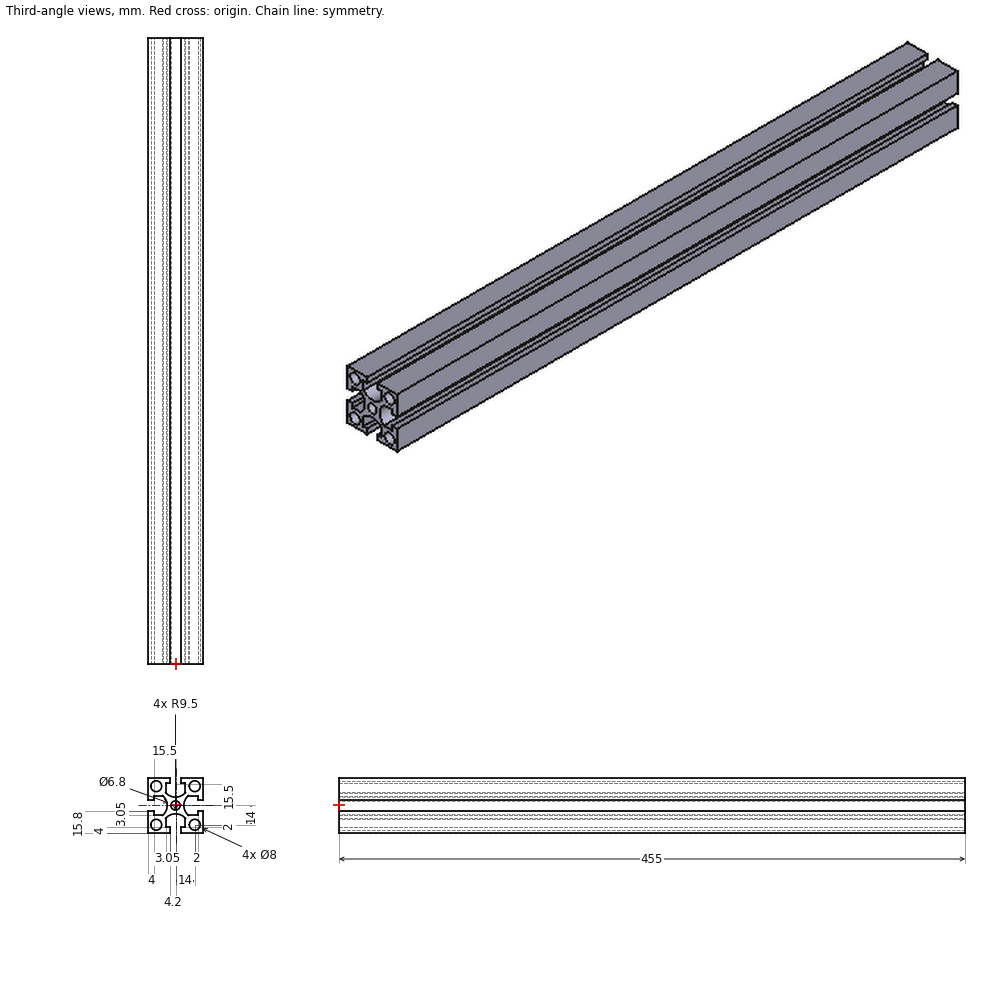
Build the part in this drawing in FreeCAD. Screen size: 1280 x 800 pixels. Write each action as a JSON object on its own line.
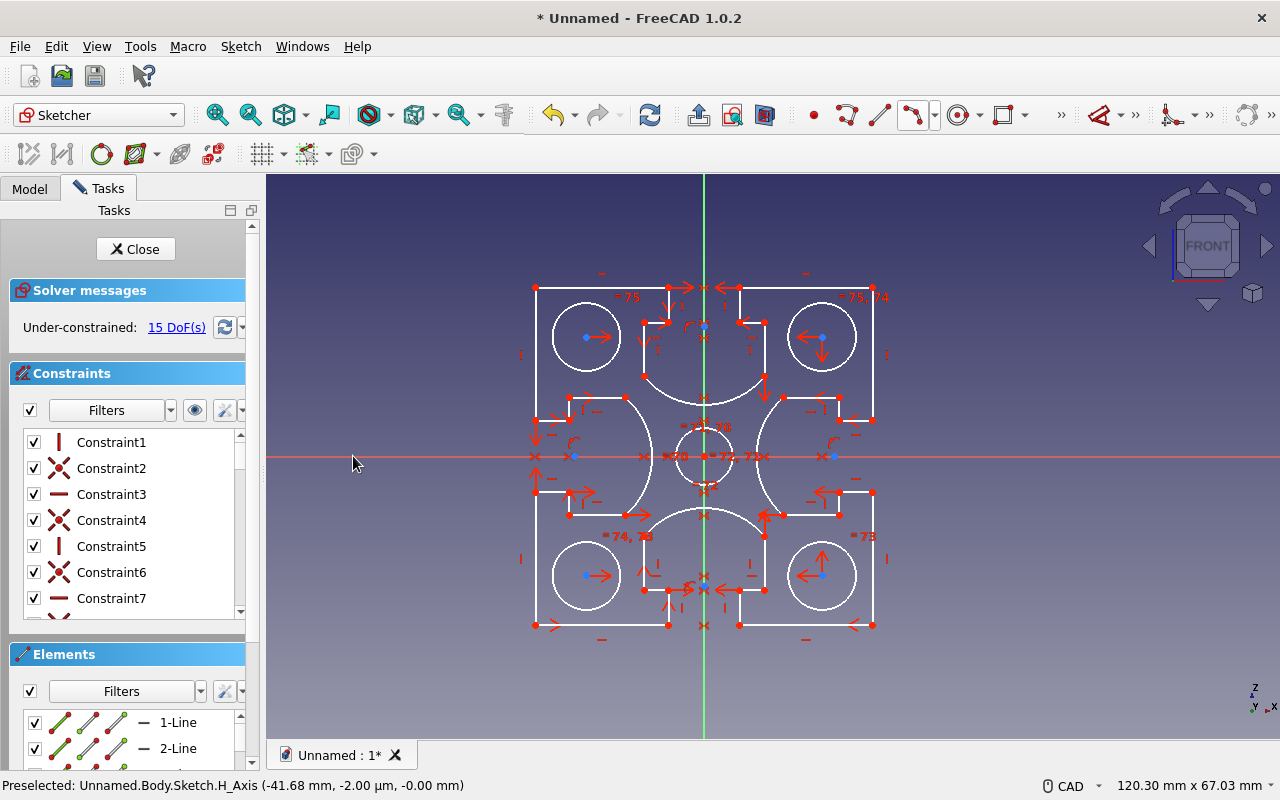
{"action": "left_click", "coordinate": [1098, 116]}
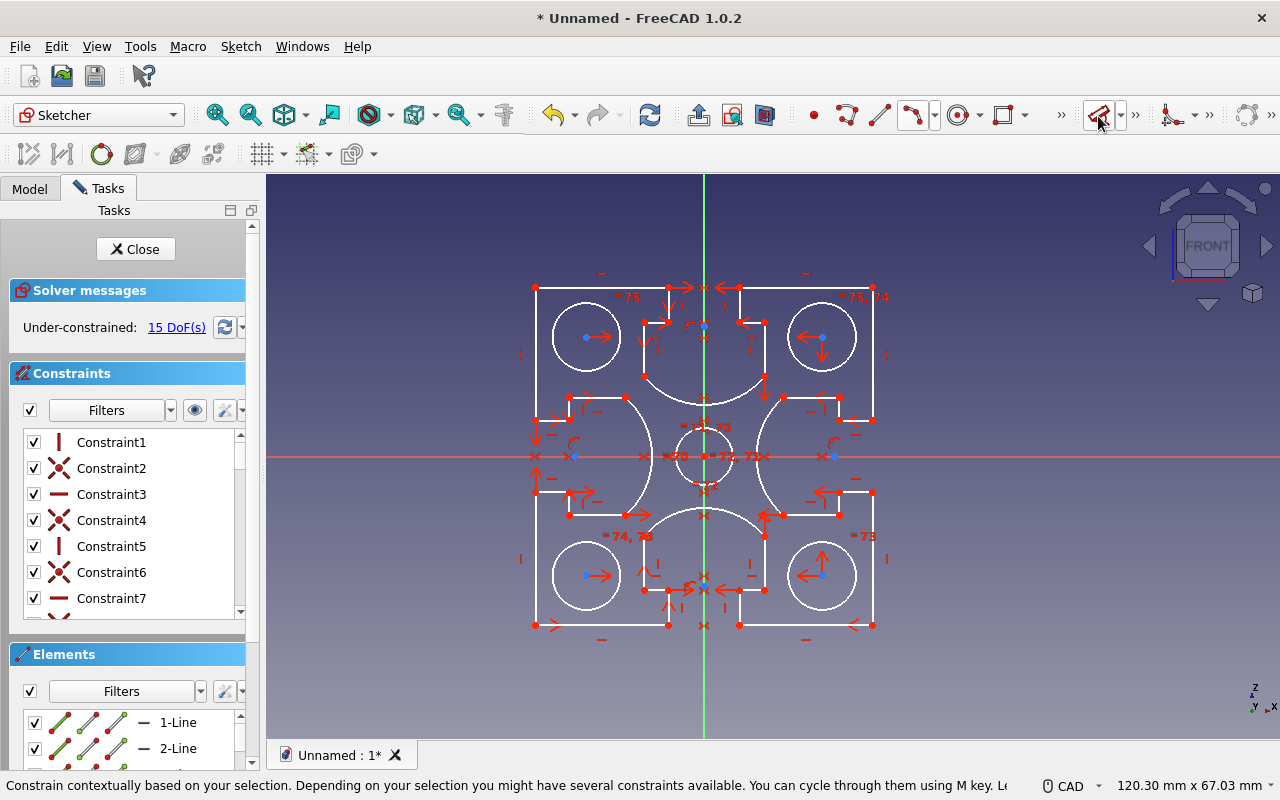
{"action": "left_click", "coordinate": [648, 483]}
{"action": "left_click", "coordinate": [678, 494]}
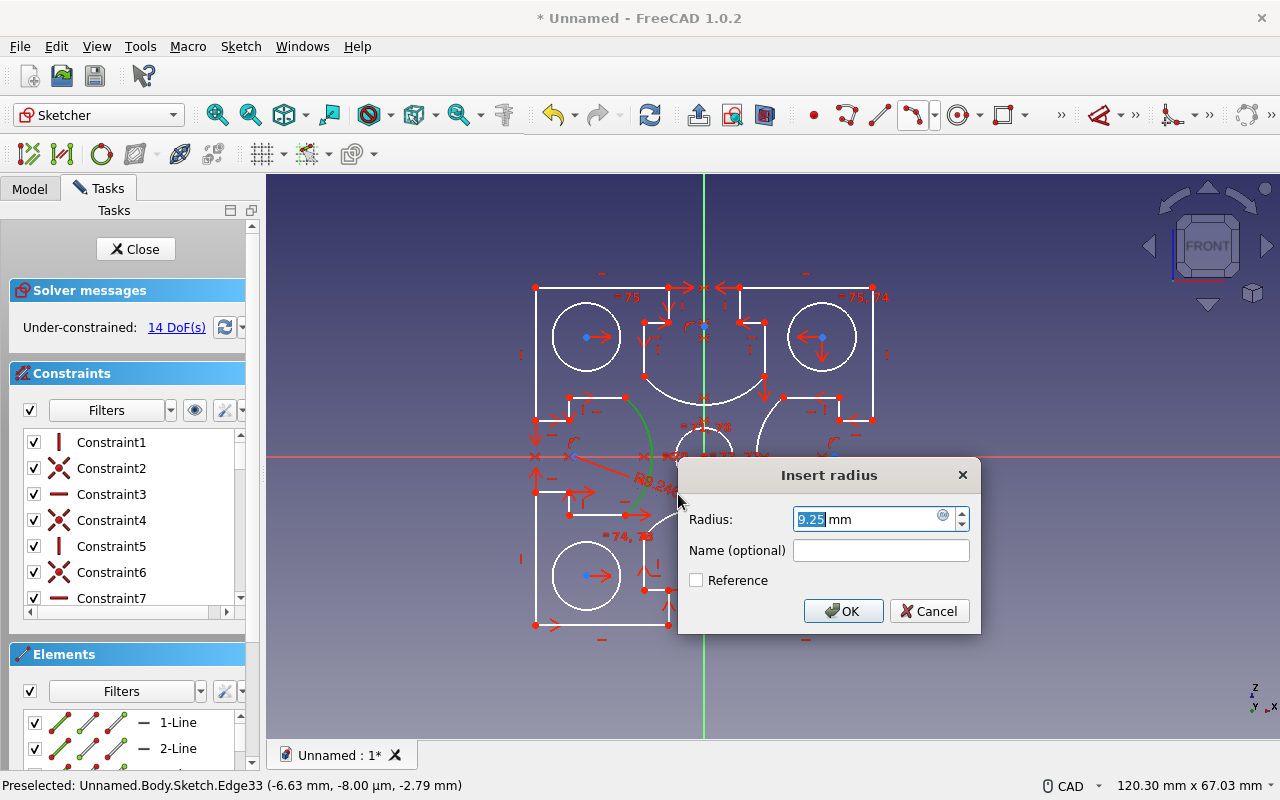
{"action": "type", "text": "9.5"}
{"action": "key", "text": "Return"}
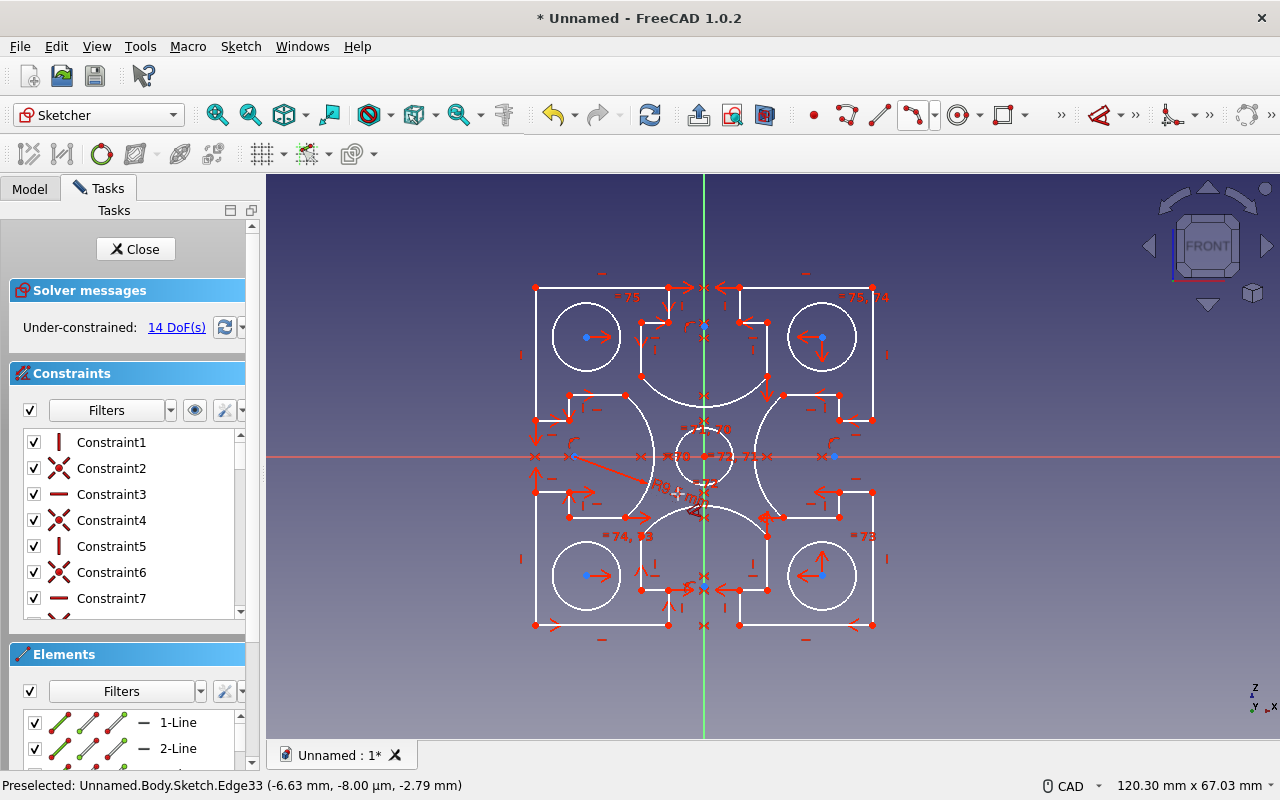
{"action": "left_click", "coordinate": [846, 552]}
{"action": "left_click", "coordinate": [887, 590]}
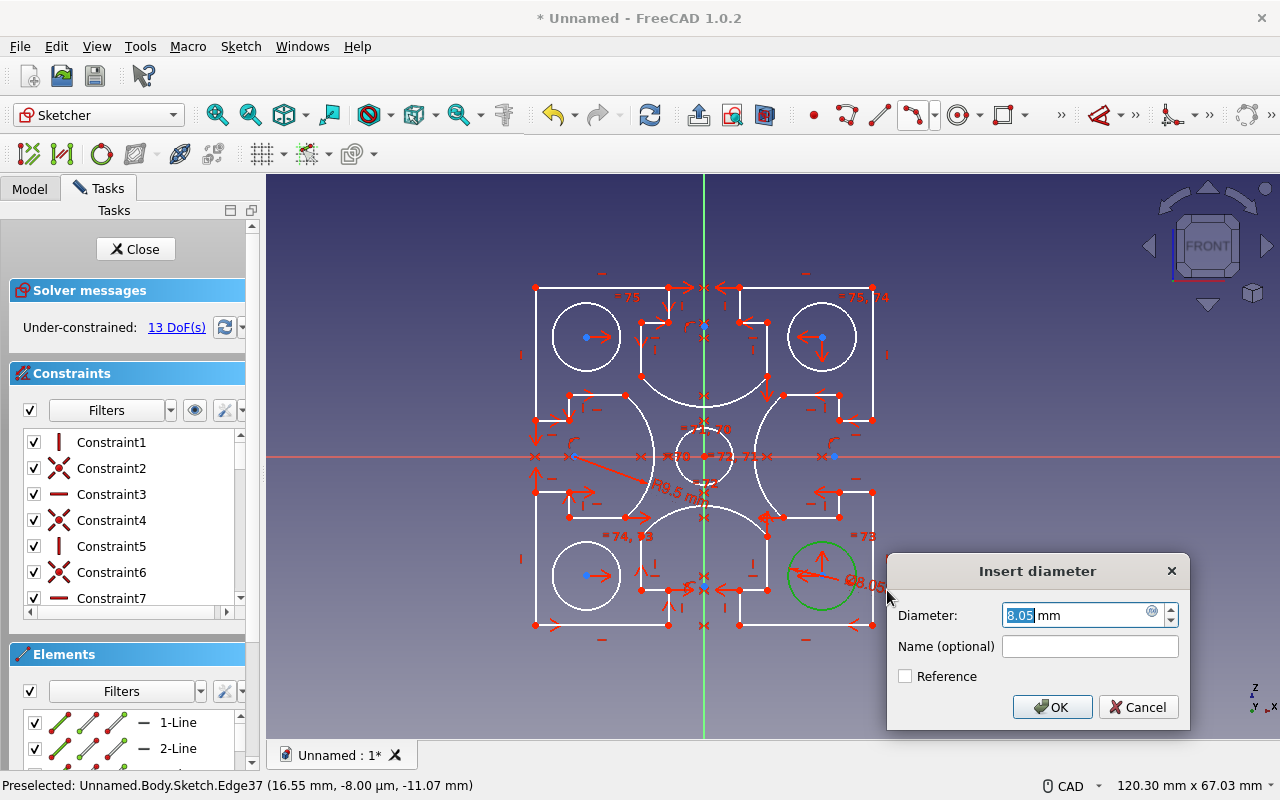
{"action": "type", "text": "8"}
{"action": "key", "text": "Return"}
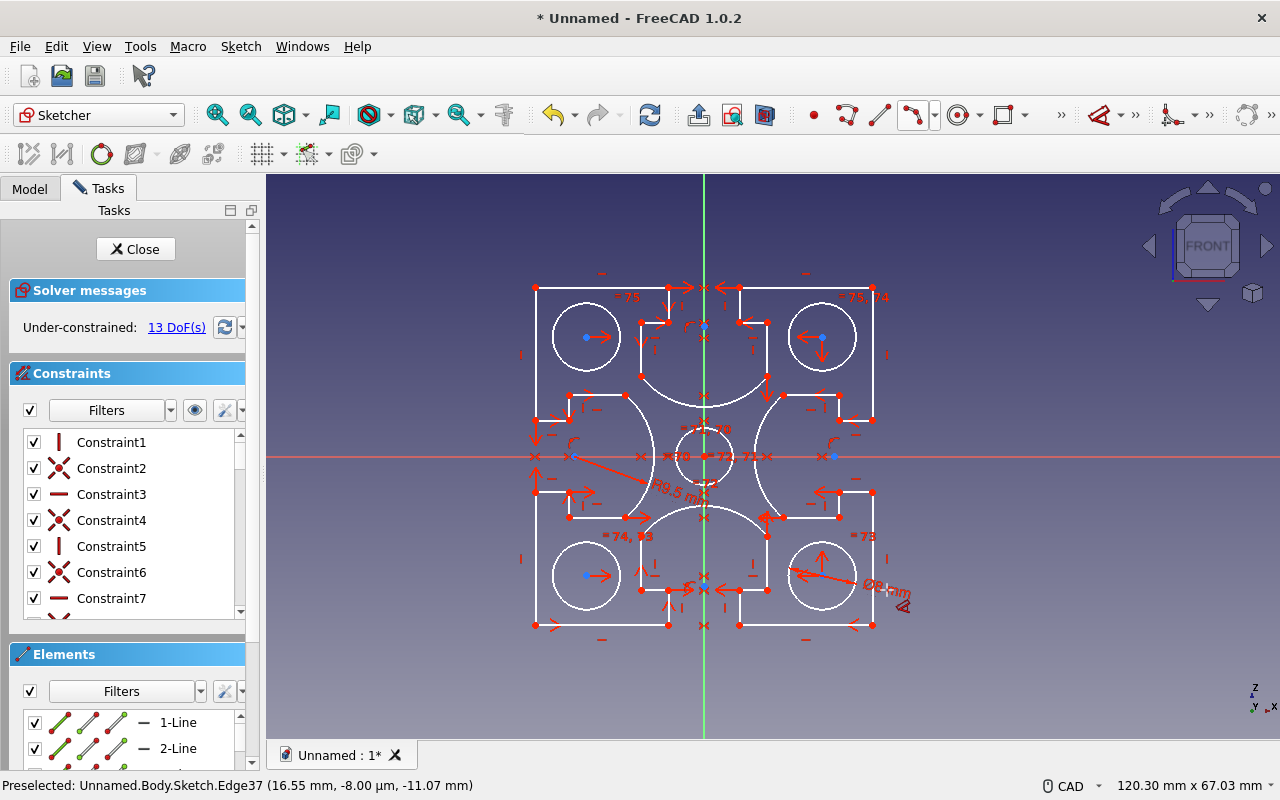
{"action": "left_click", "coordinate": [724, 436]}
{"action": "left_click", "coordinate": [746, 413]}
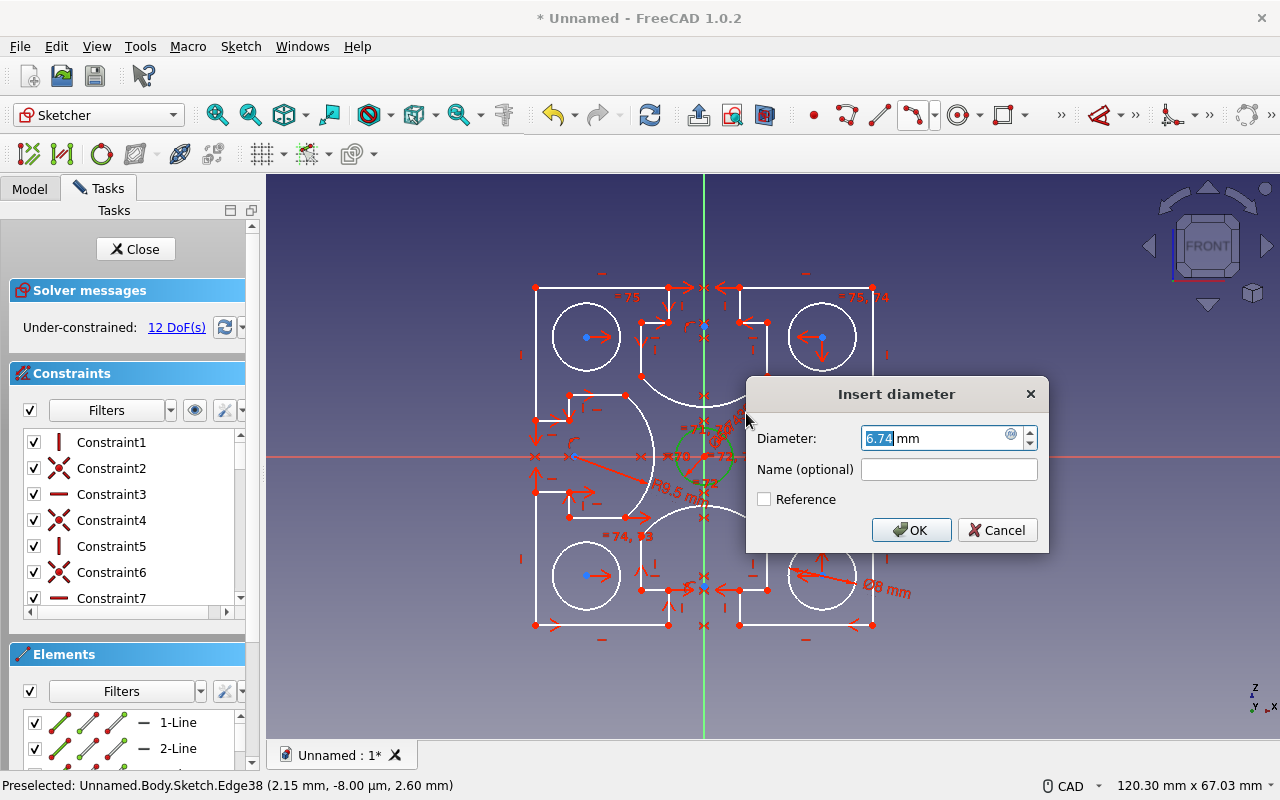
{"action": "type", "text": "6.8"}
{"action": "key", "text": "Return"}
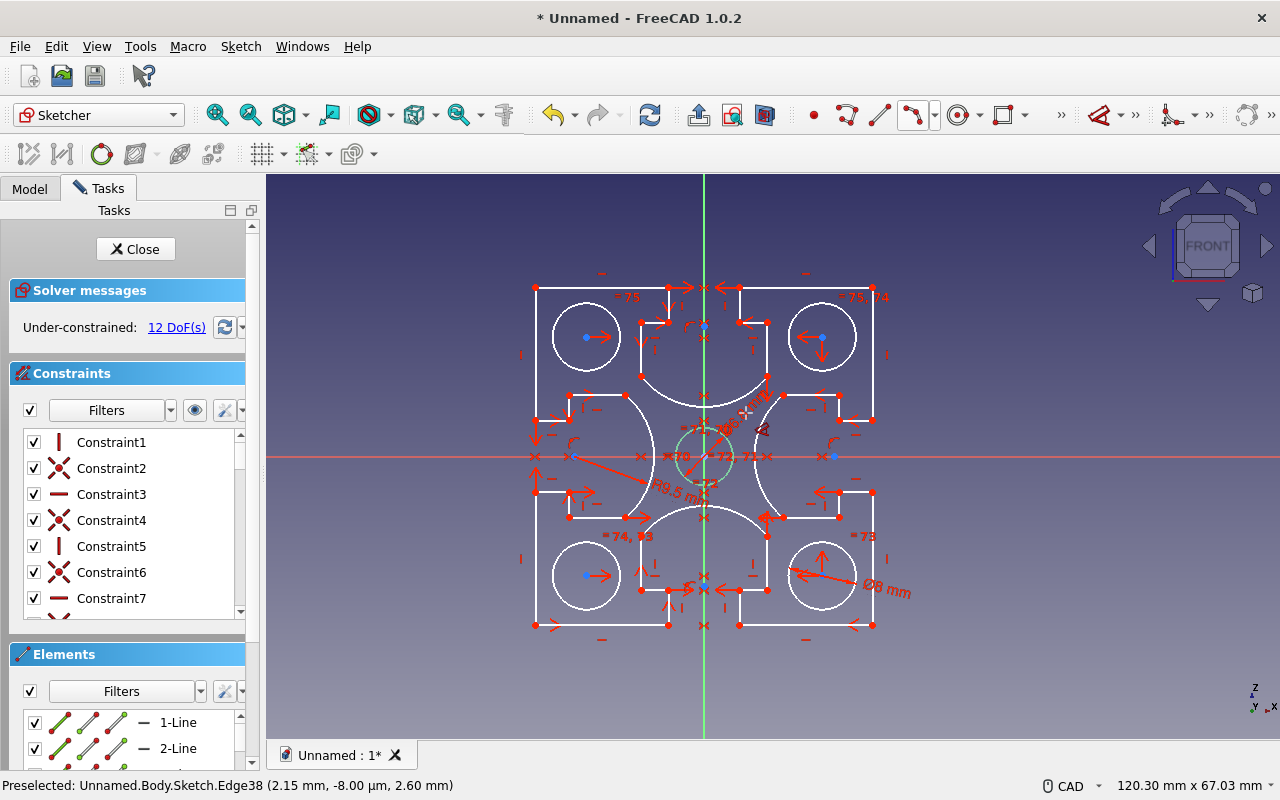
{"action": "scroll", "coordinate": [669, 601], "scroll_direction": "up", "scroll_amount": 2}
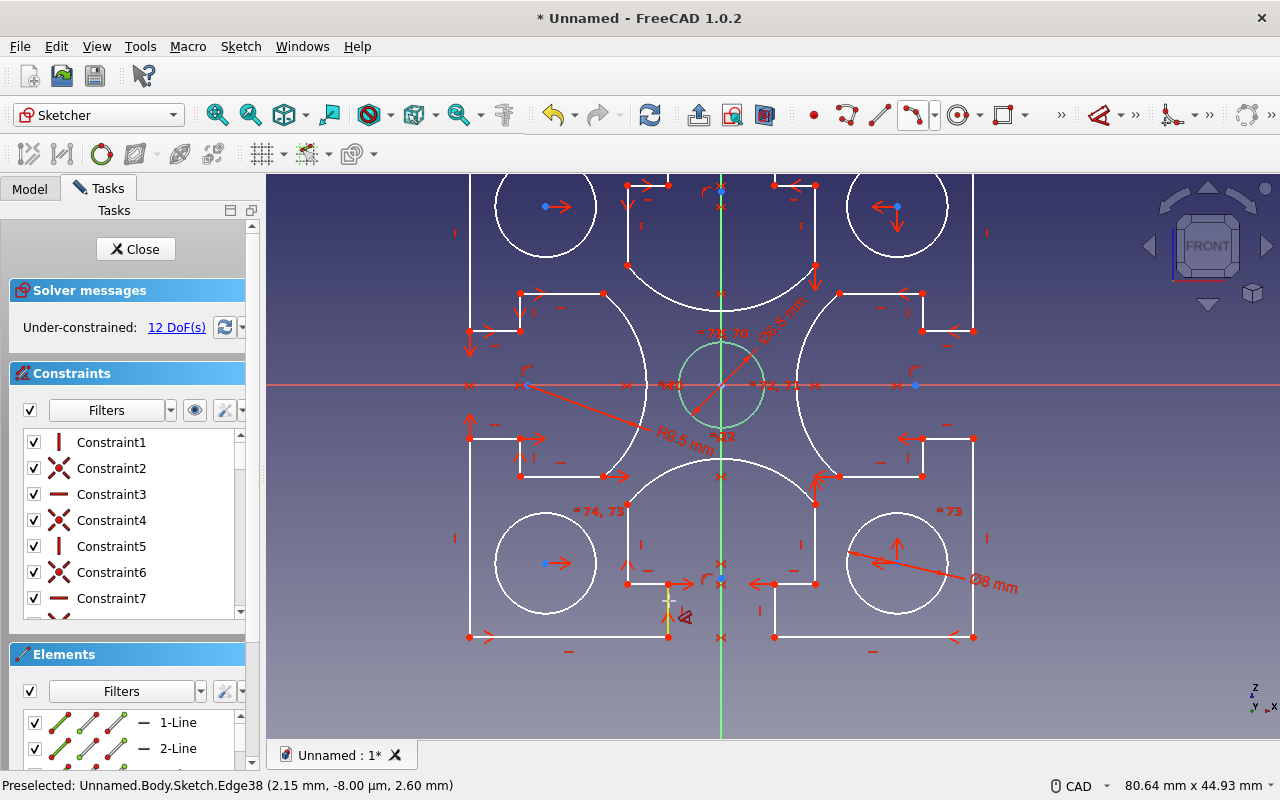
{"action": "left_click", "coordinate": [668, 600]}
{"action": "left_click", "coordinate": [634, 611]}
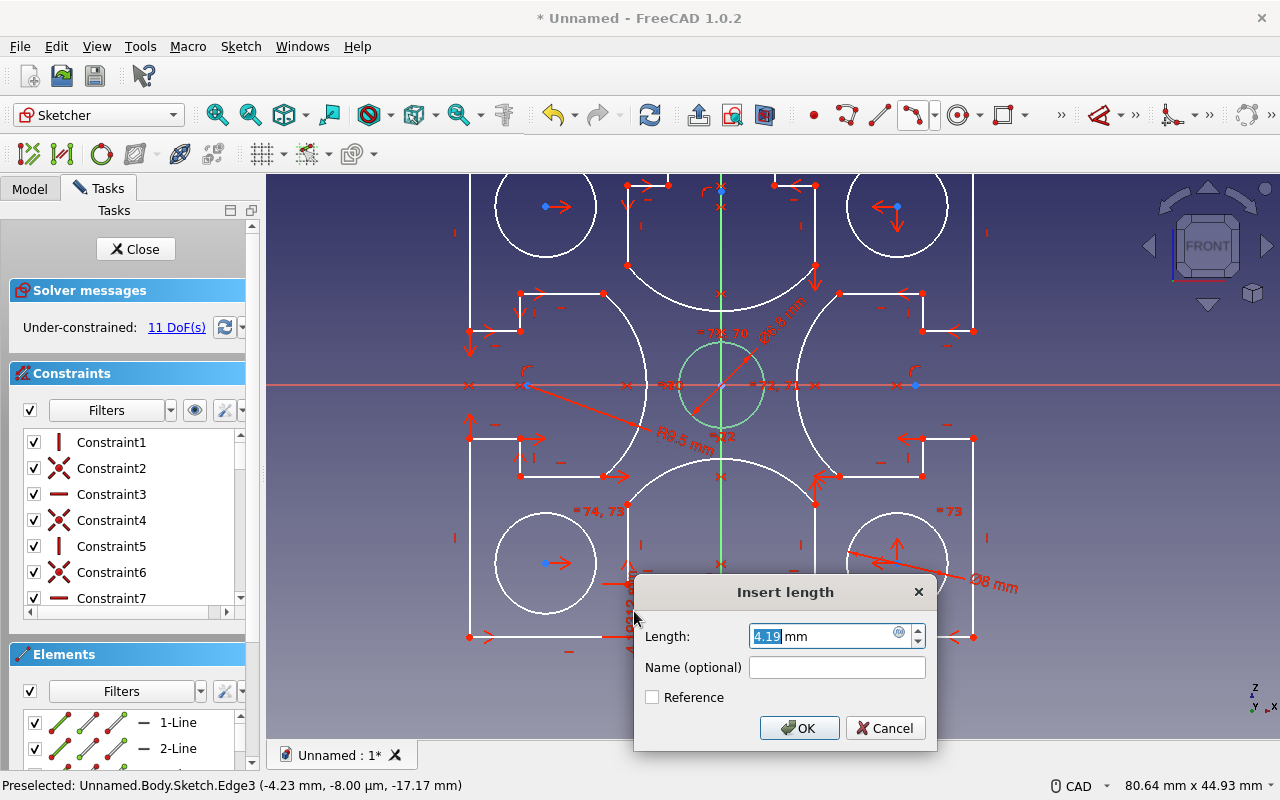
{"action": "type", "text": "4"}
{"action": "key", "text": "Return"}